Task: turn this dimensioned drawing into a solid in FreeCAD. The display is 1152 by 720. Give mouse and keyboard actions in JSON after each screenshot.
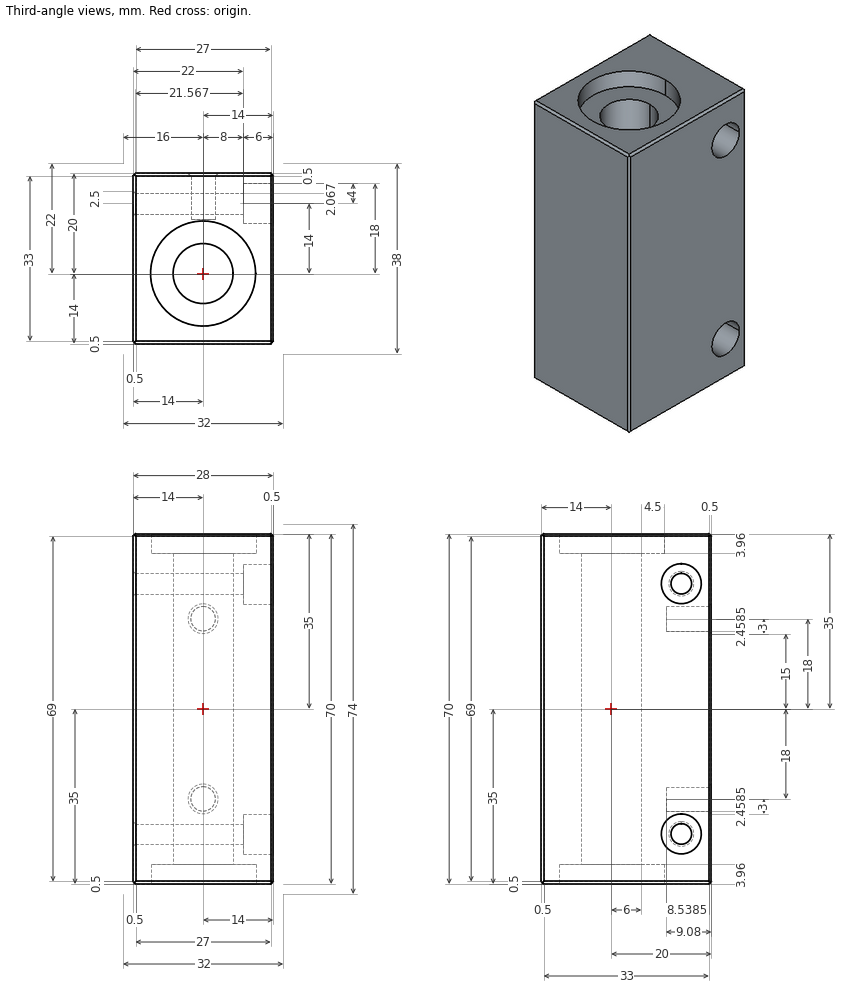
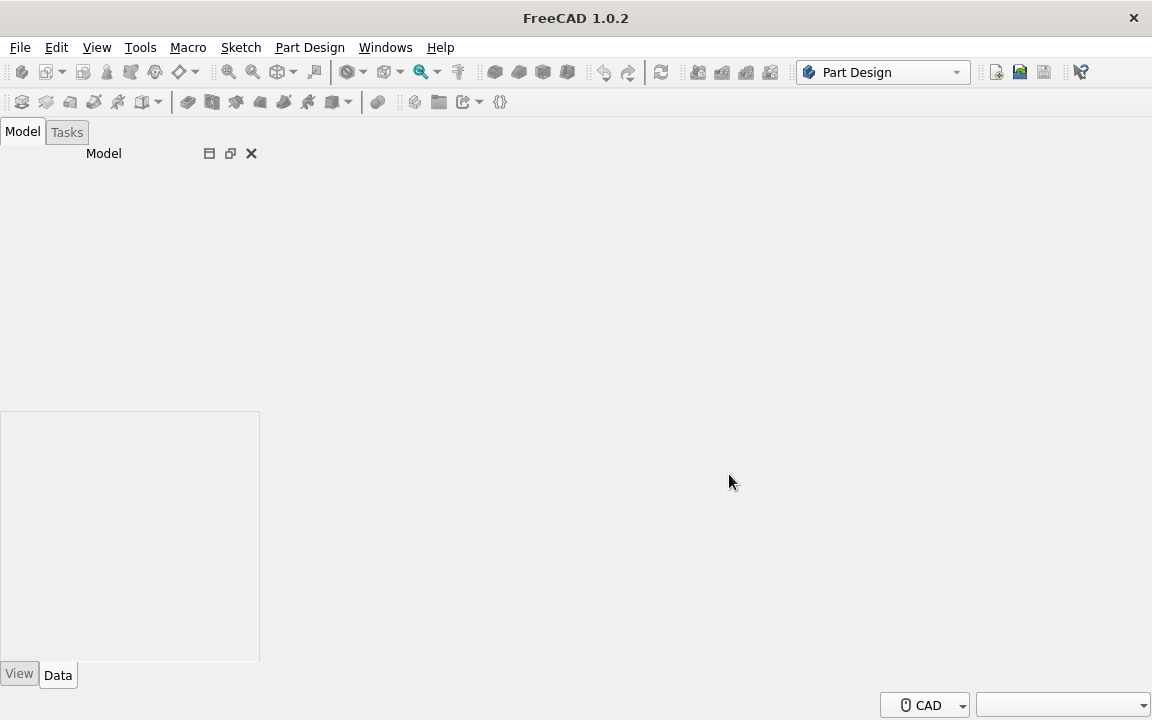
{"action": "left_click", "coordinate": [996, 72]}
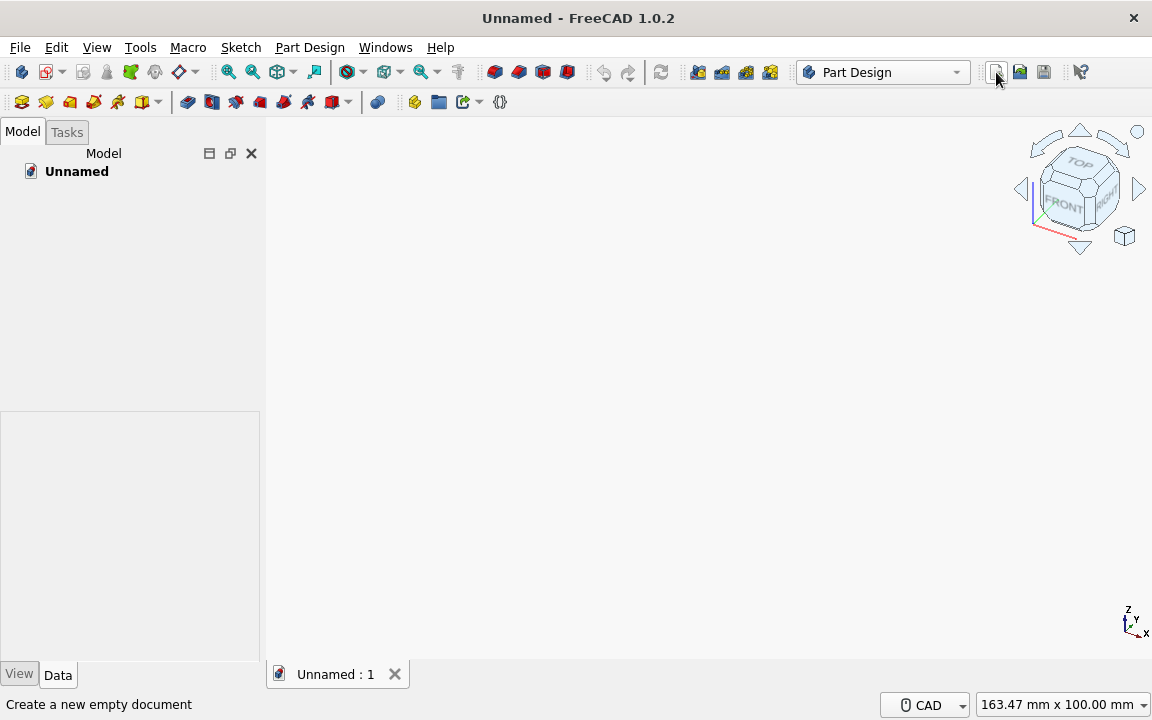
{"action": "left_click", "coordinate": [46, 72]}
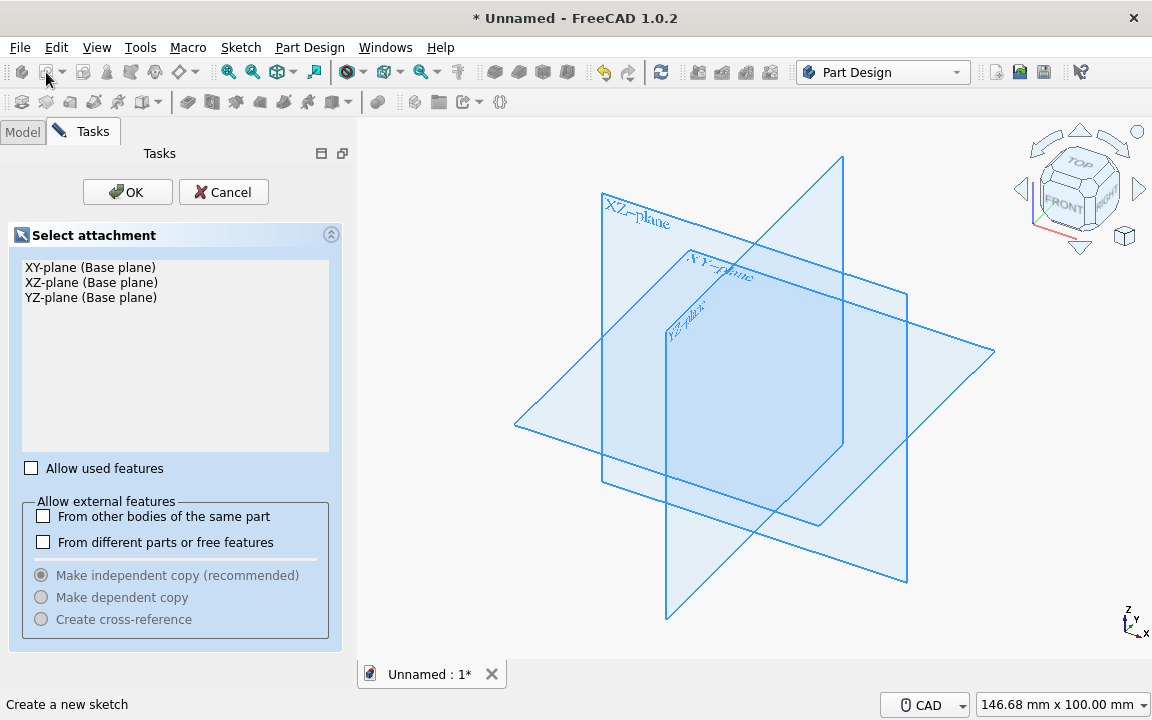
{"action": "left_click", "coordinate": [82, 298]}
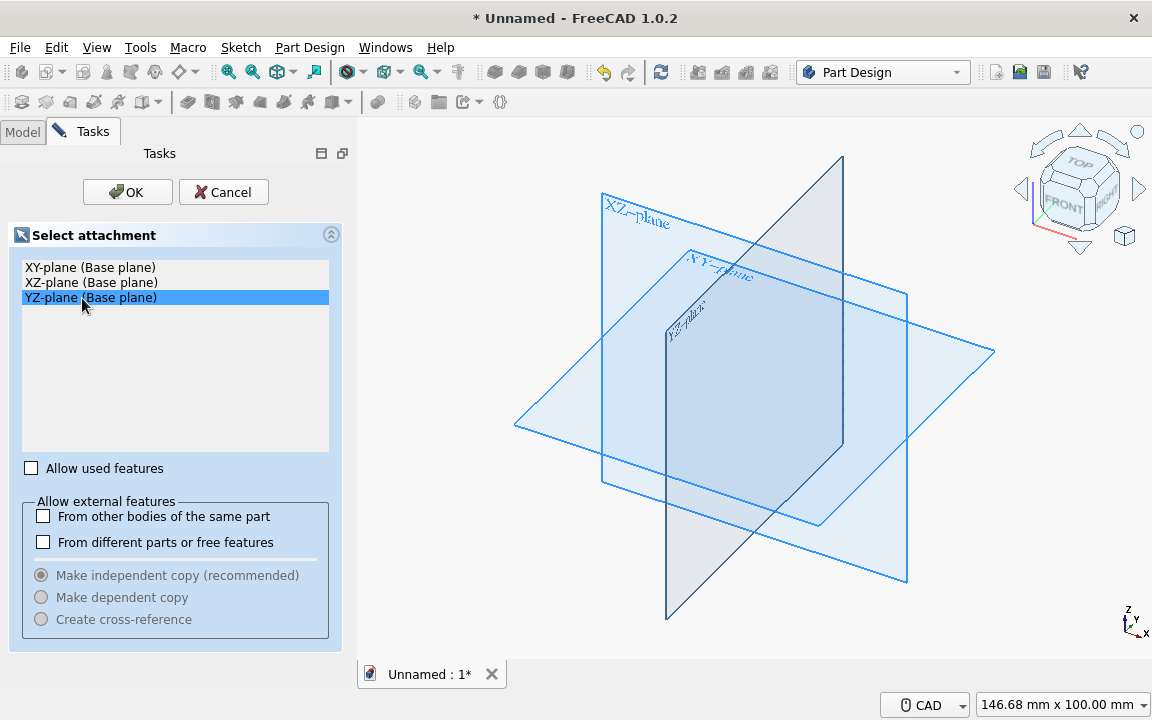
{"action": "left_click", "coordinate": [128, 192]}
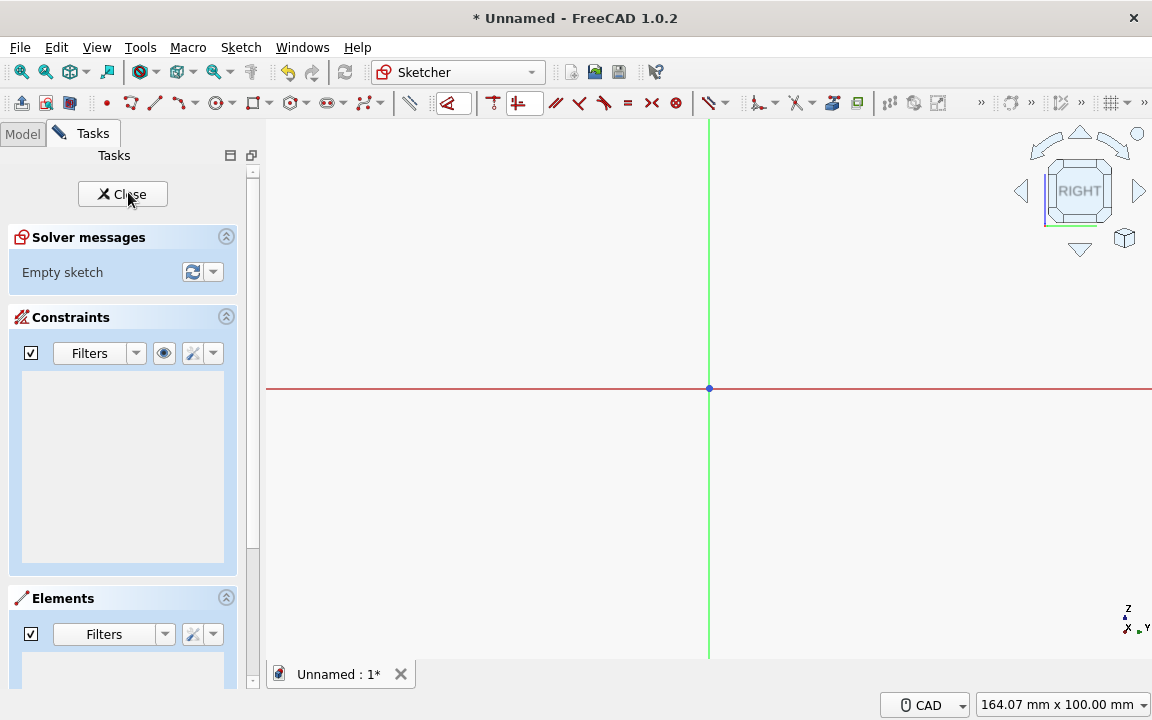
{"action": "left_click", "coordinate": [132, 104]}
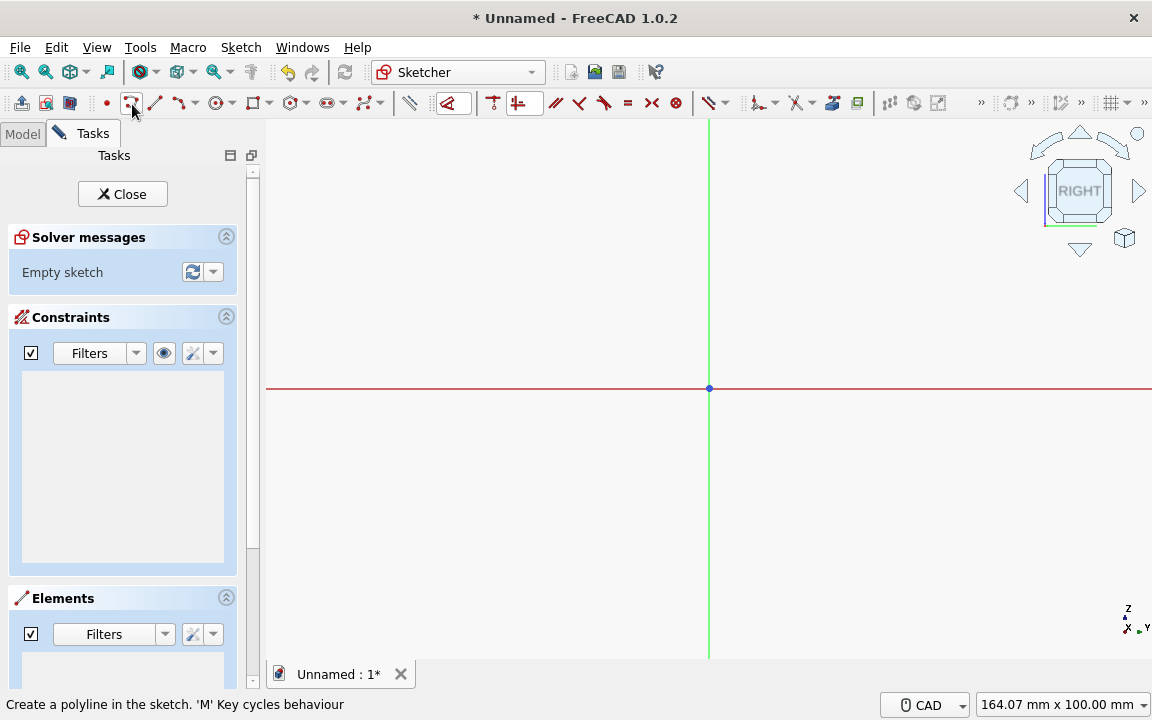
{"action": "left_click", "coordinate": [633, 203]}
{"action": "left_click", "coordinate": [633, 575]}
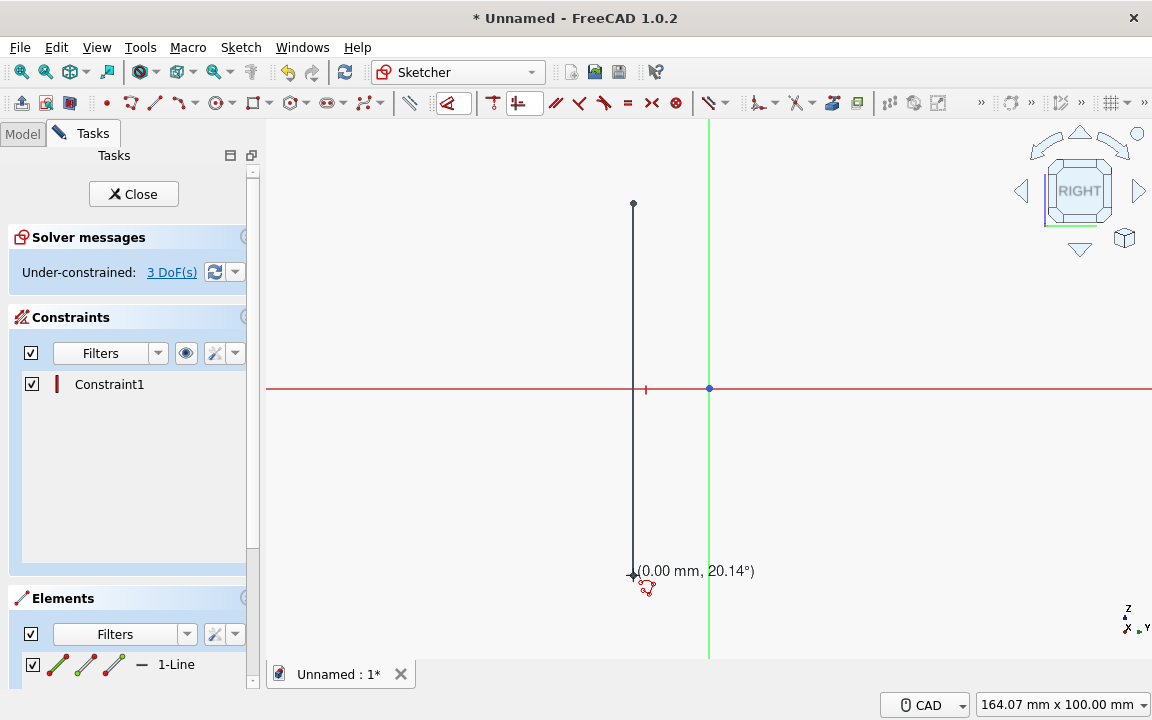
{"action": "scroll", "coordinate": [636, 578], "scroll_direction": "up", "scroll_amount": 8}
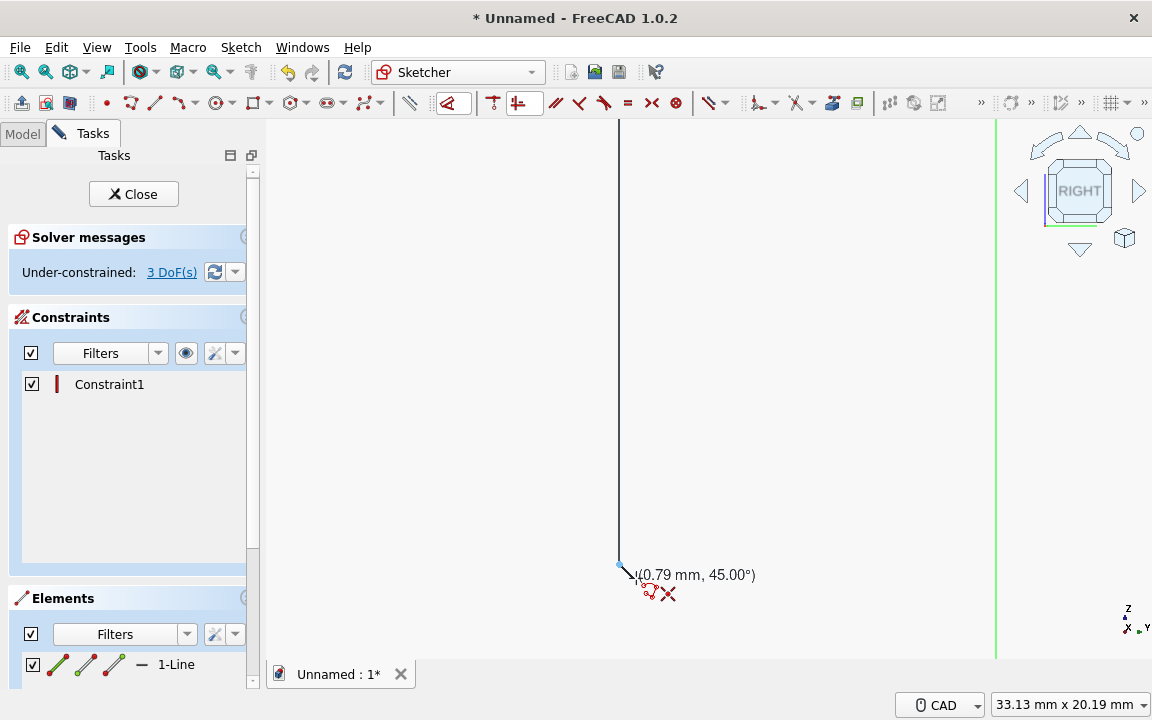
{"action": "left_click", "coordinate": [635, 575]}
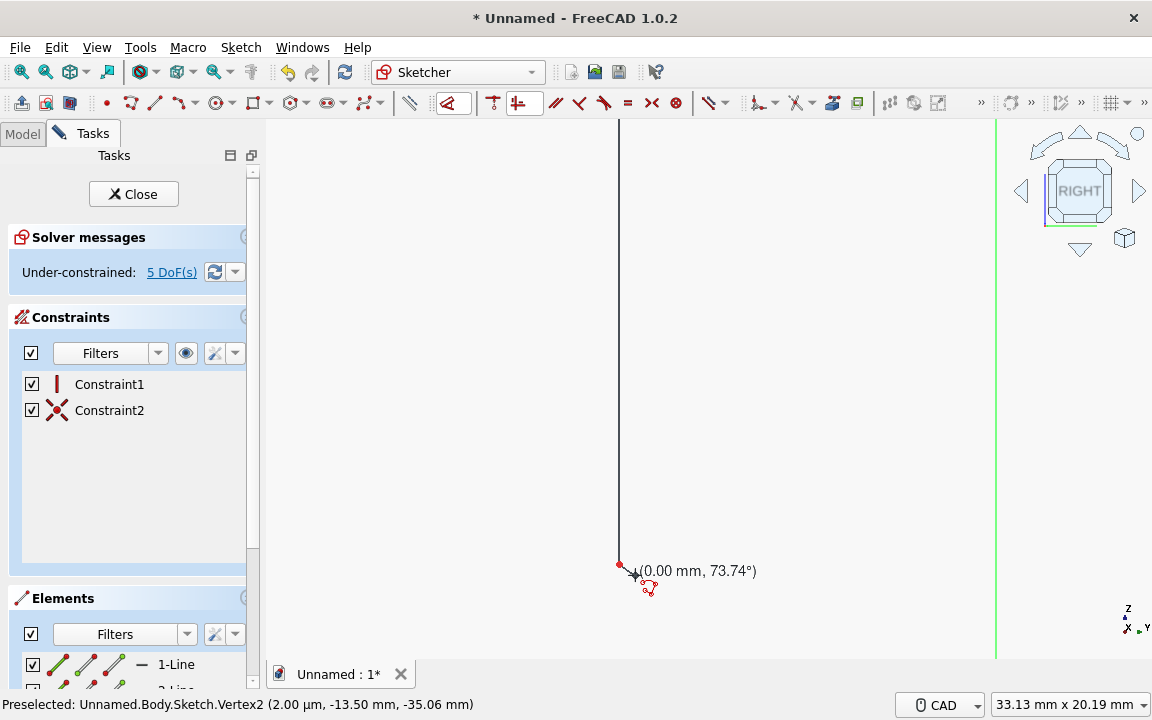
{"action": "scroll", "coordinate": [554, 538], "scroll_direction": "down", "scroll_amount": 9}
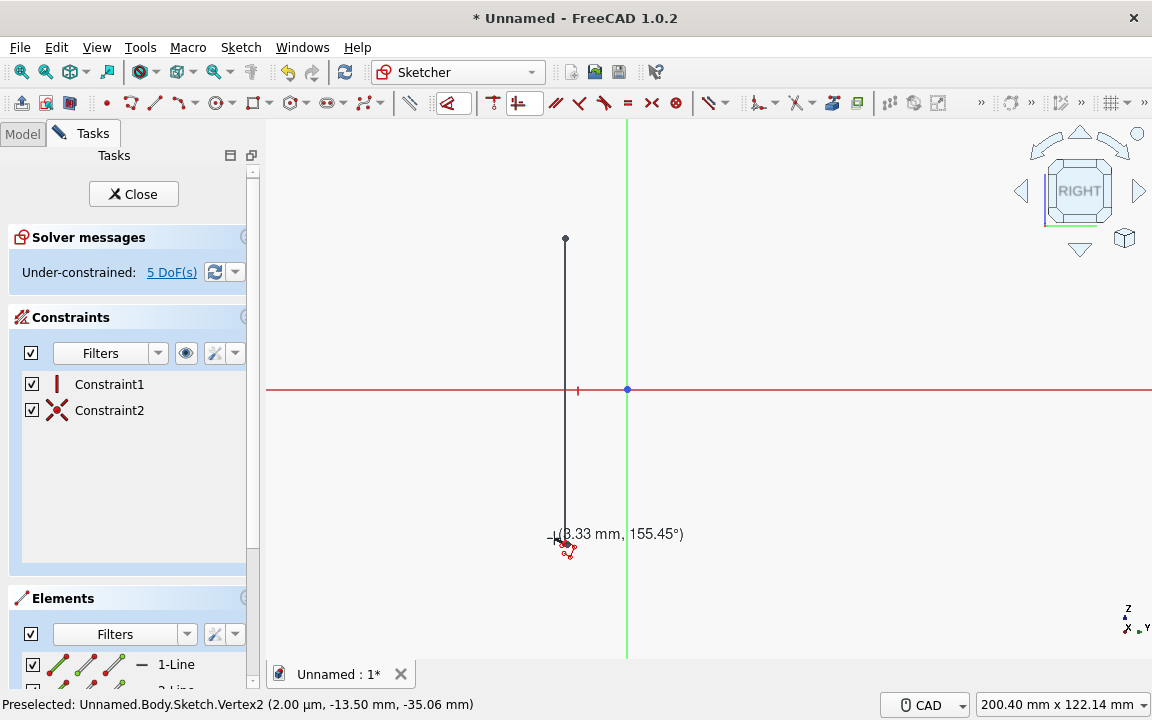
{"action": "left_click", "coordinate": [714, 545]}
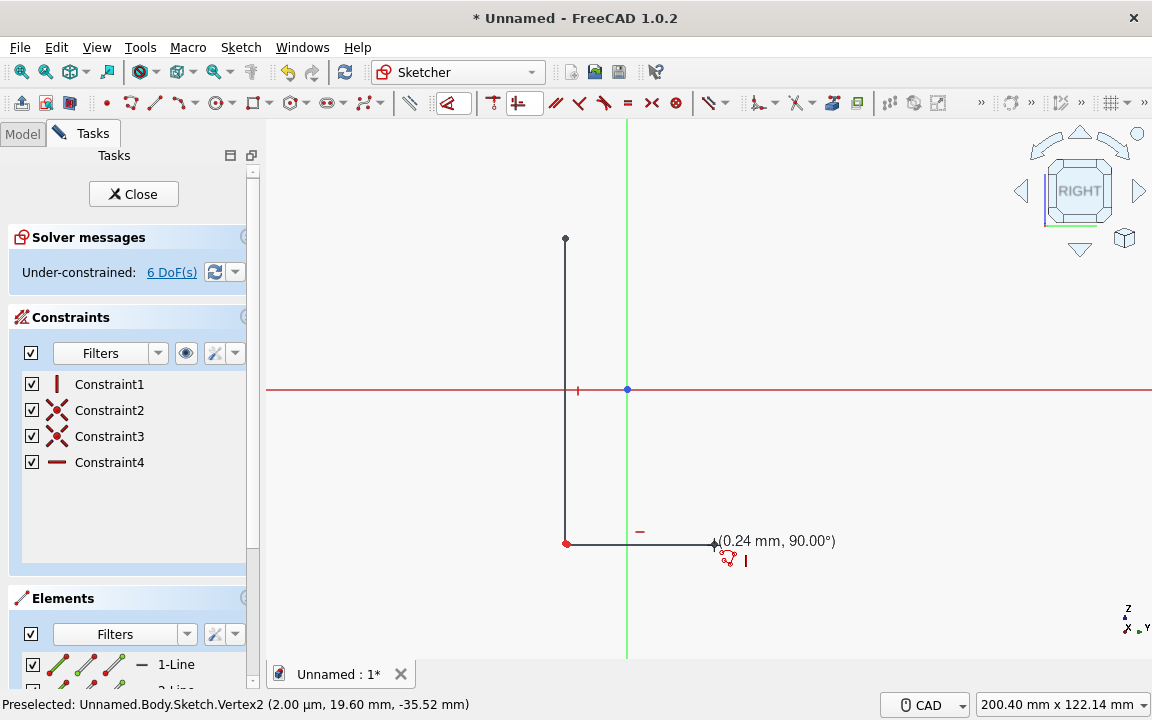
{"action": "scroll", "coordinate": [716, 542], "scroll_direction": "up", "scroll_amount": 9}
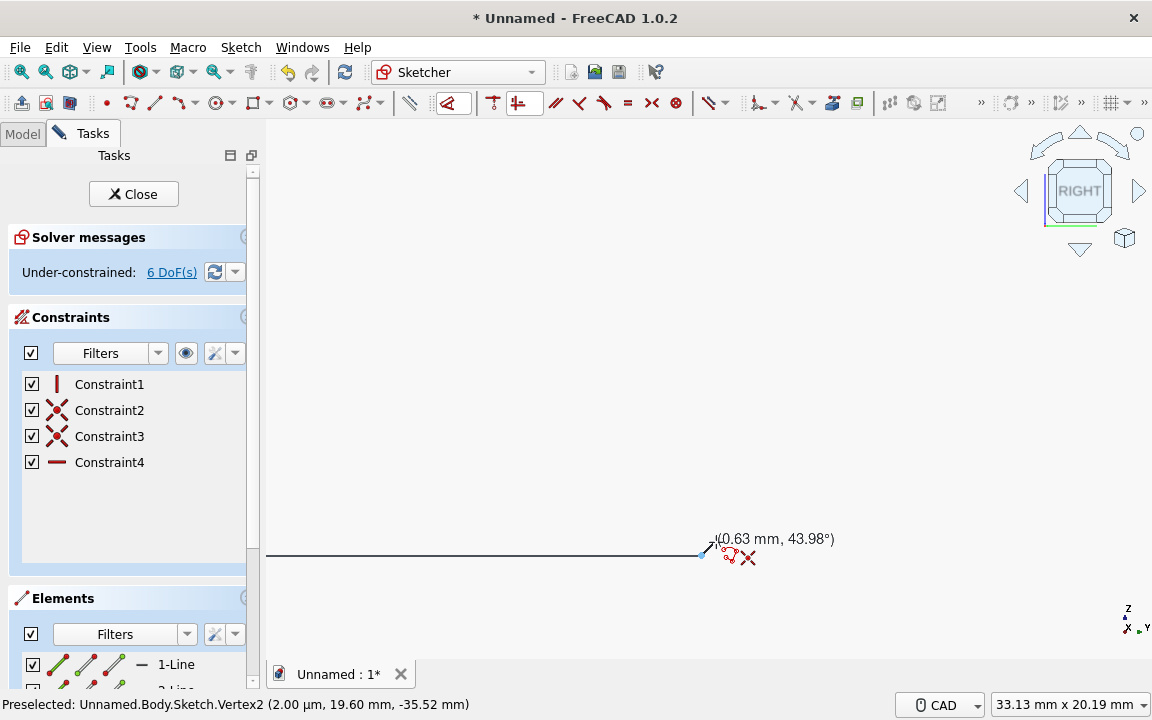
{"action": "left_click", "coordinate": [712, 541]}